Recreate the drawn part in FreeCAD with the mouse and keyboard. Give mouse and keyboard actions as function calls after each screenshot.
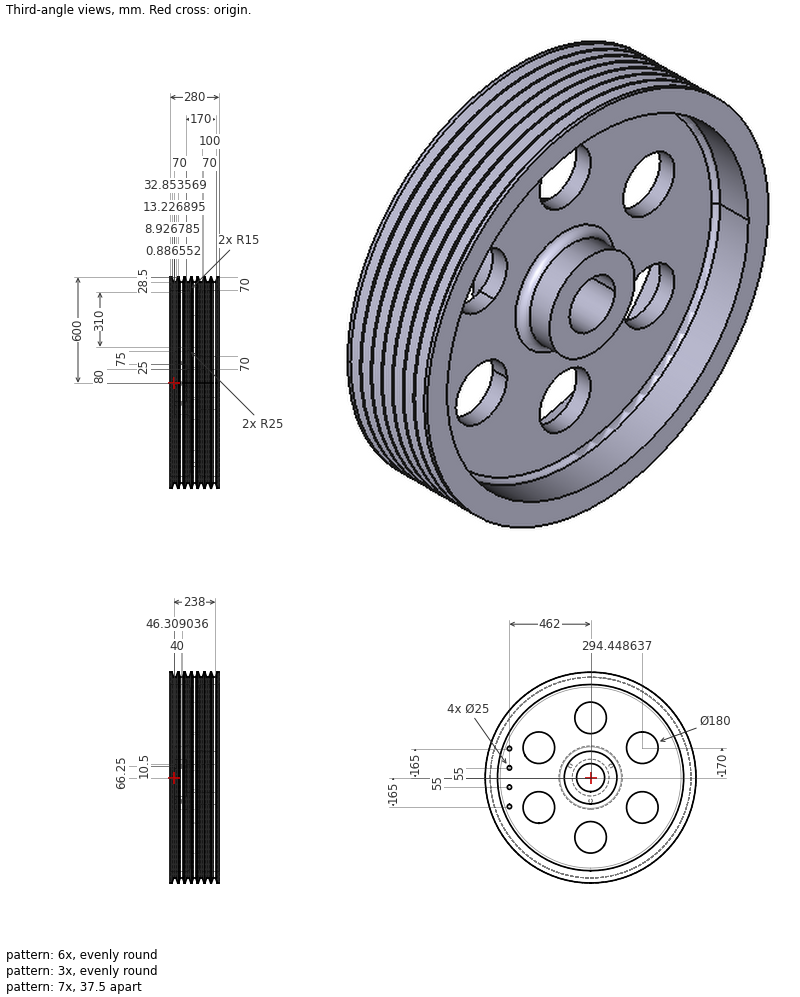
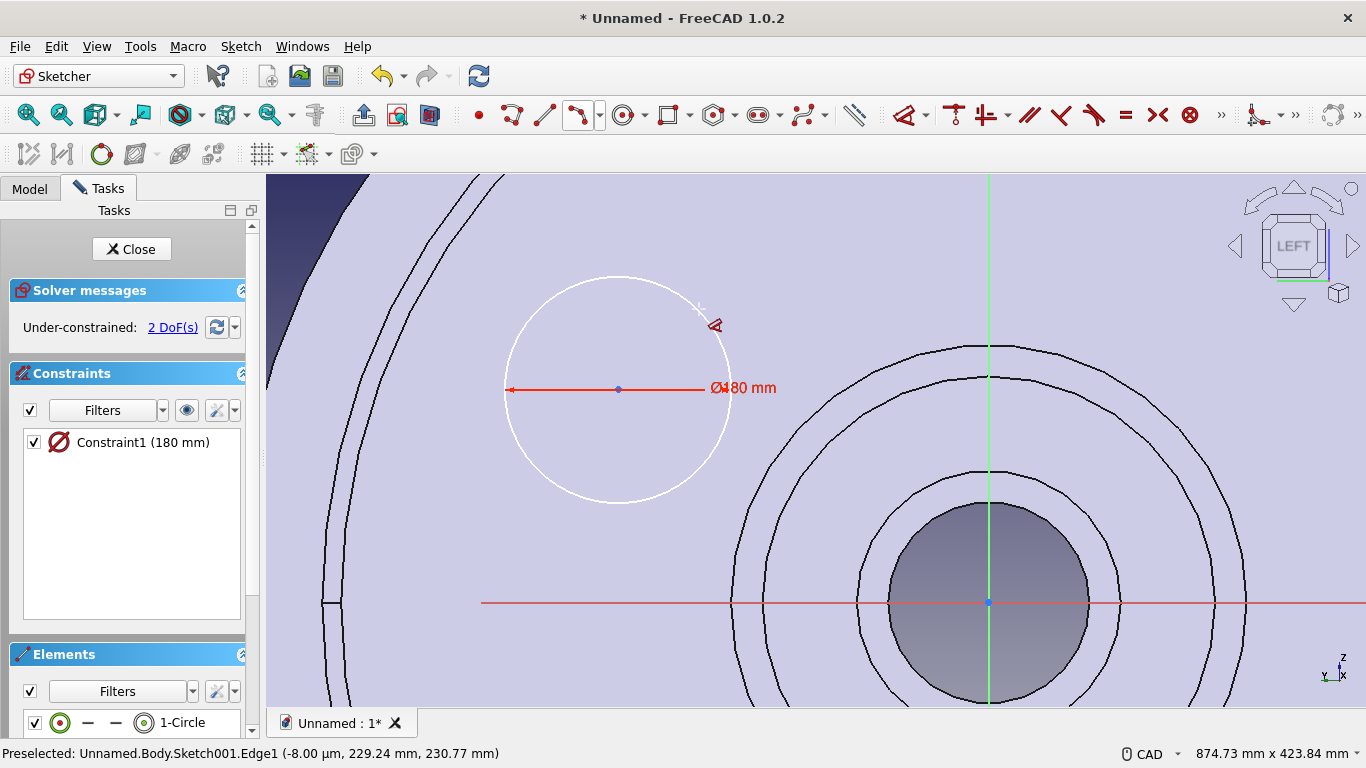
click(618, 390)
click(1023, 496)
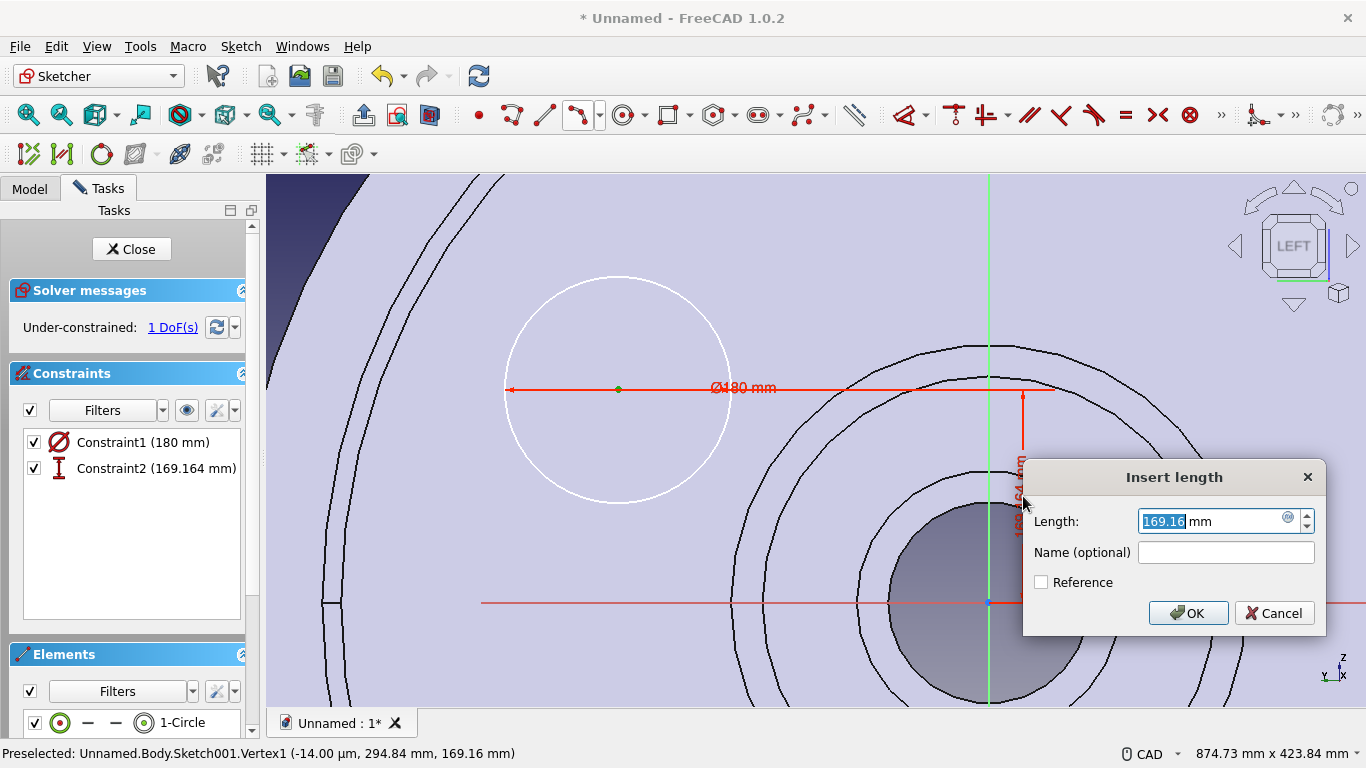
text(170)
key(Return)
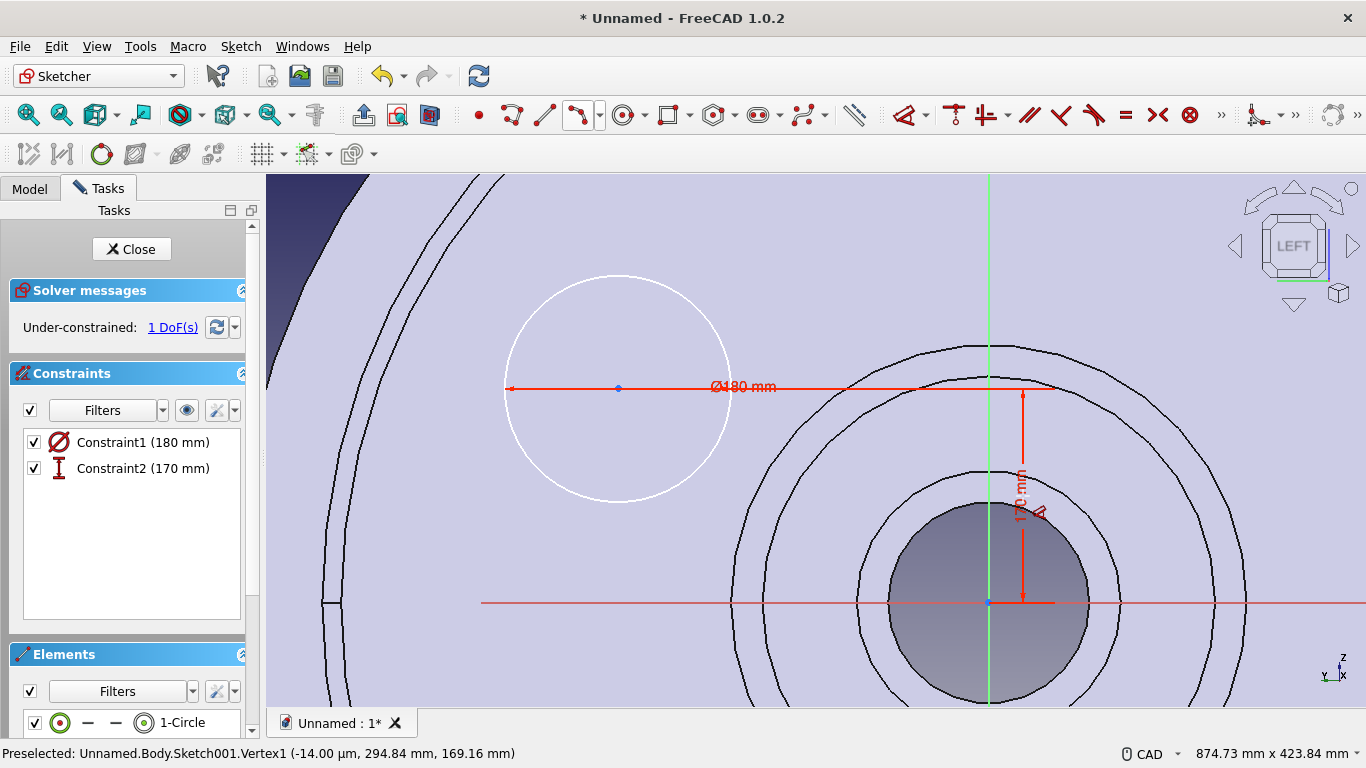
click(618, 389)
click(803, 637)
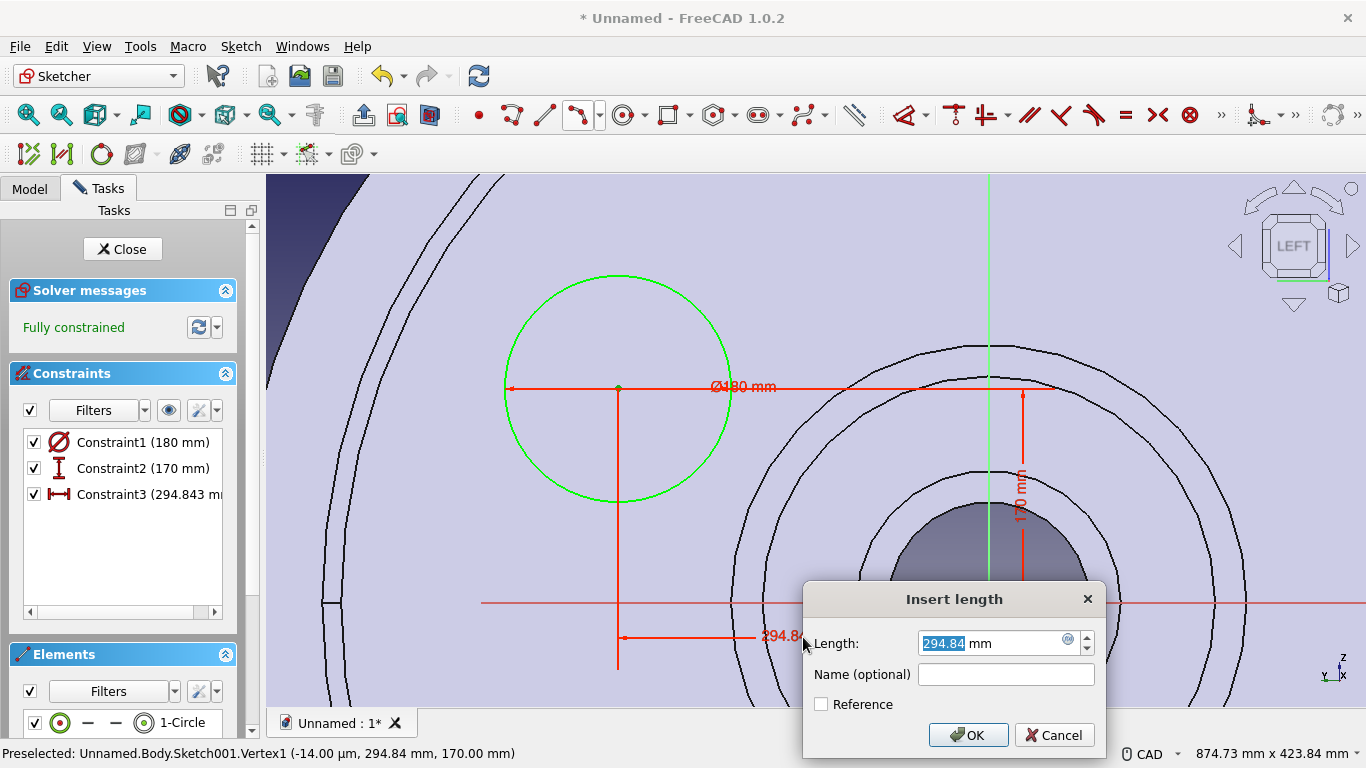
text(294.448637)
key(Return)
key(Escape)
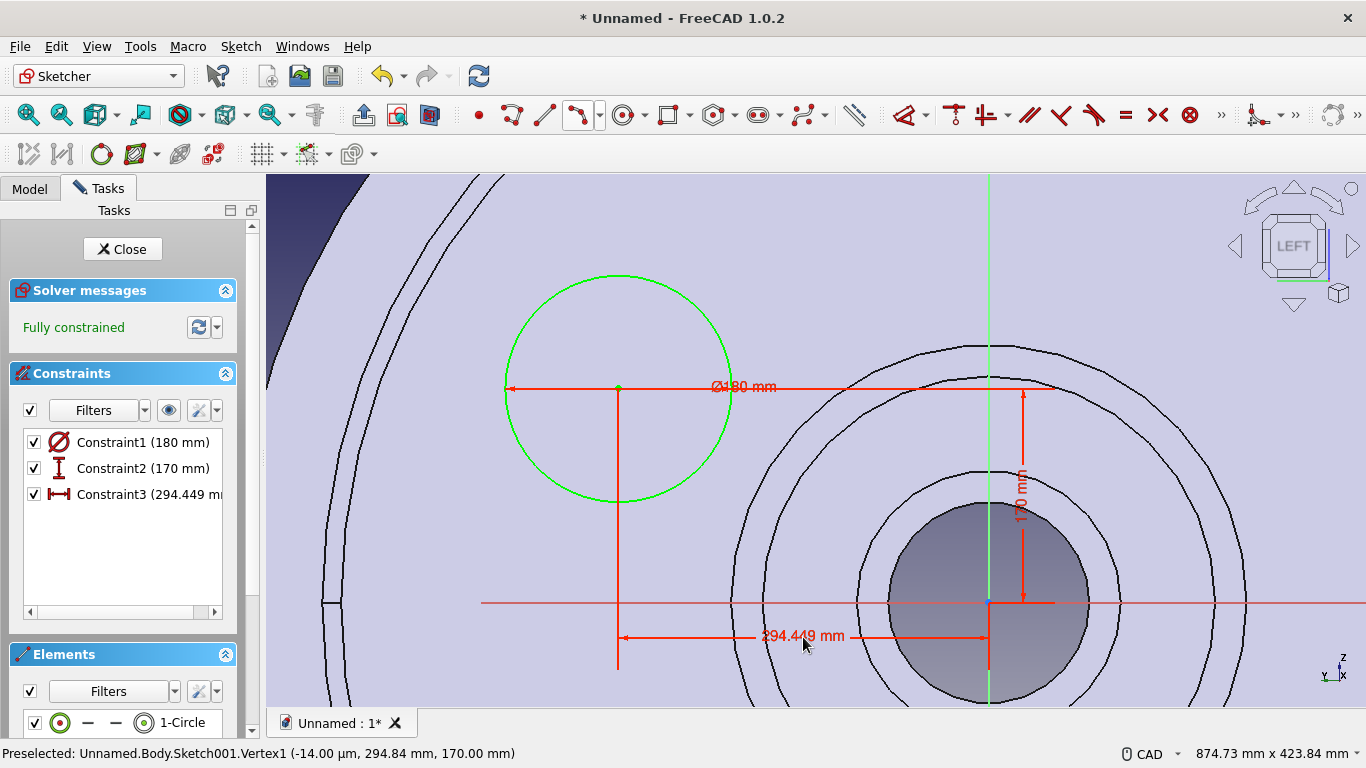
click(123, 249)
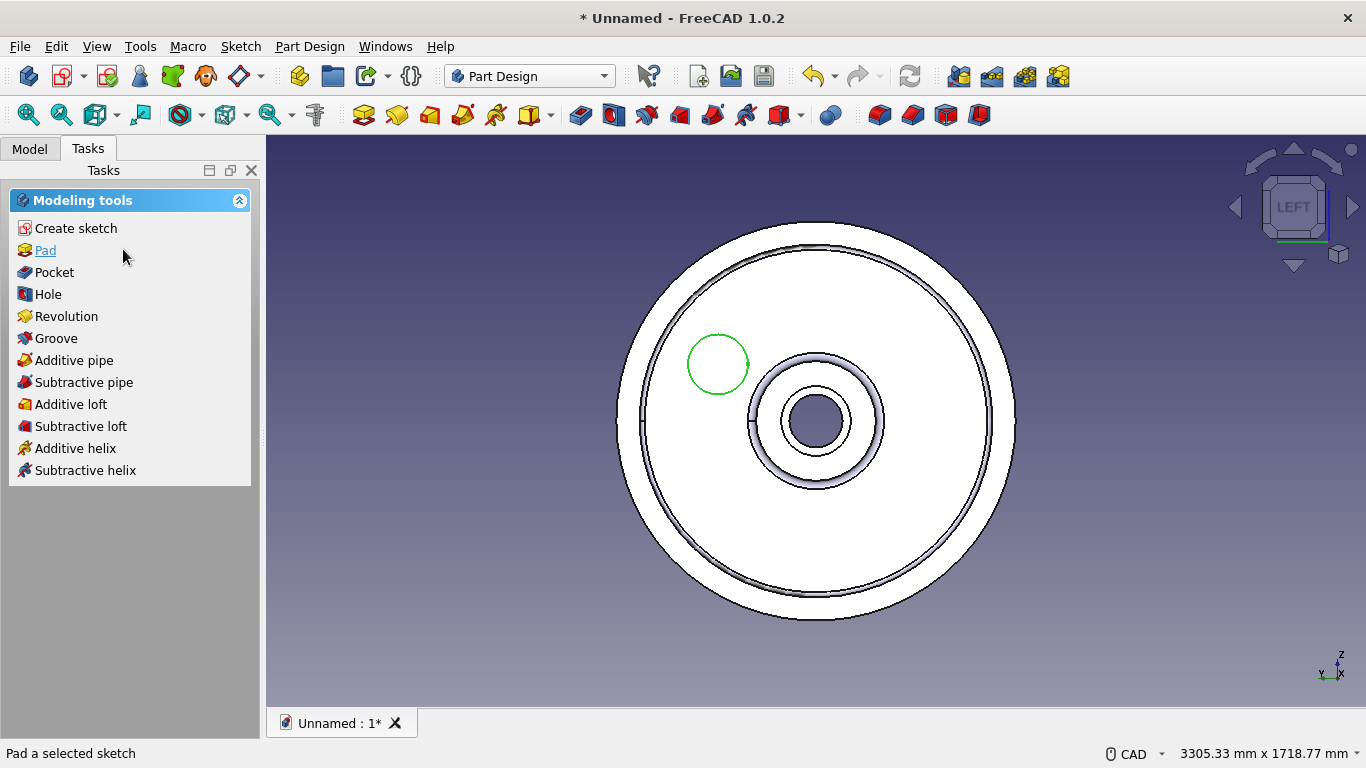
click(581, 116)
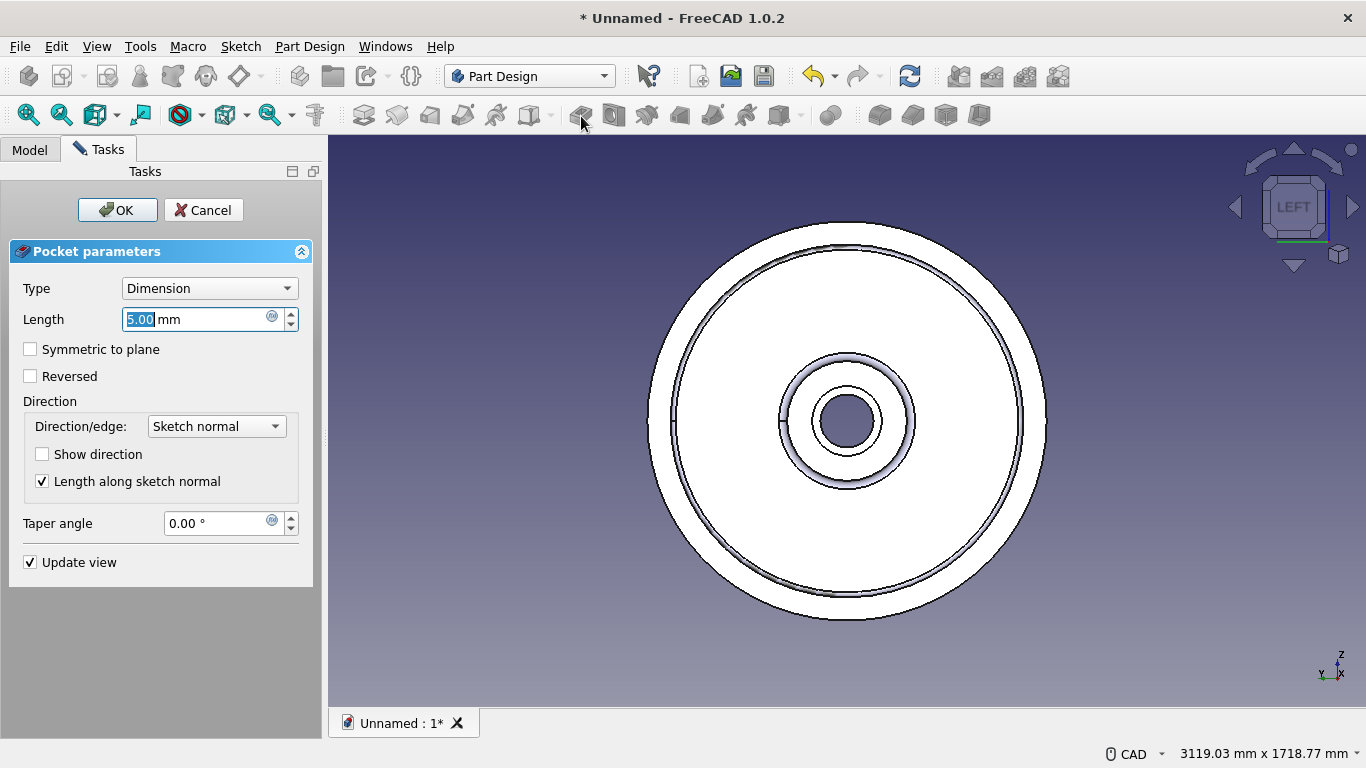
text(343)
key(Tab)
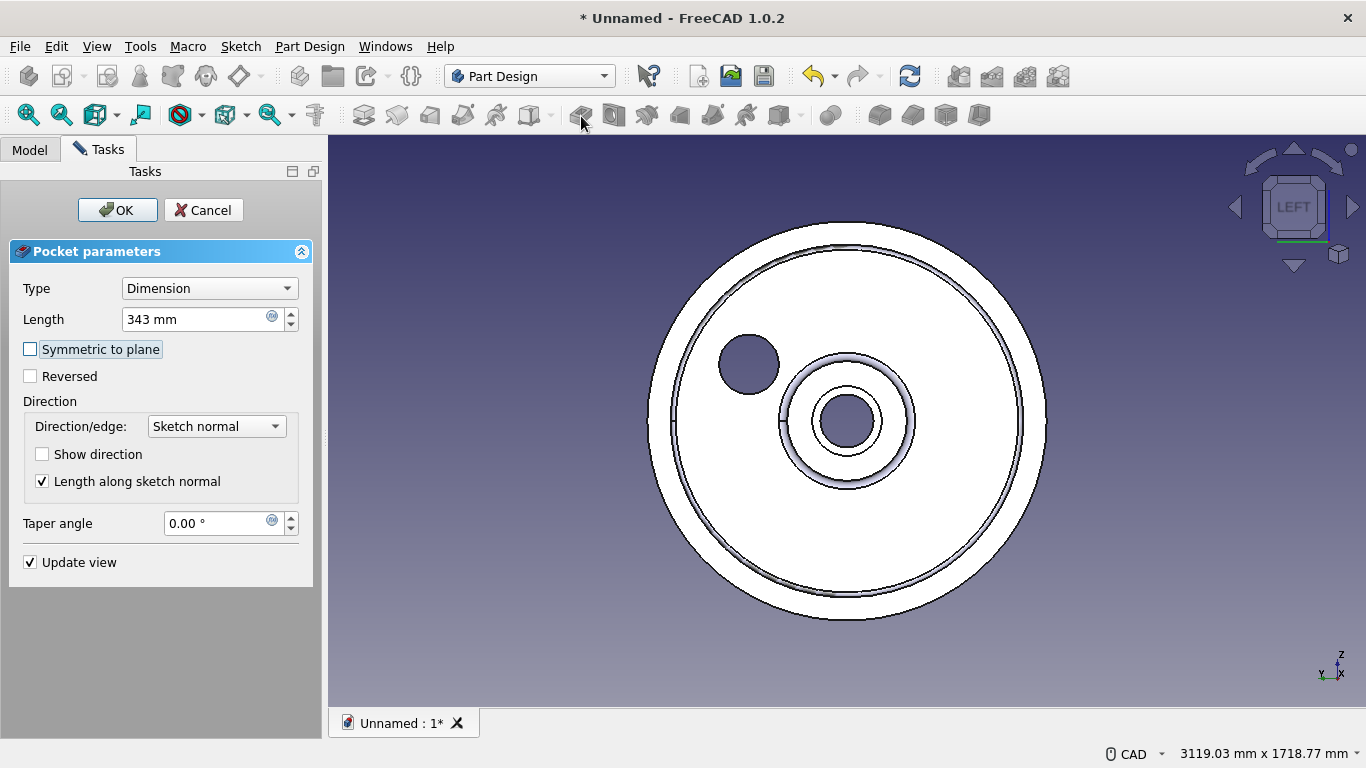
click(118, 210)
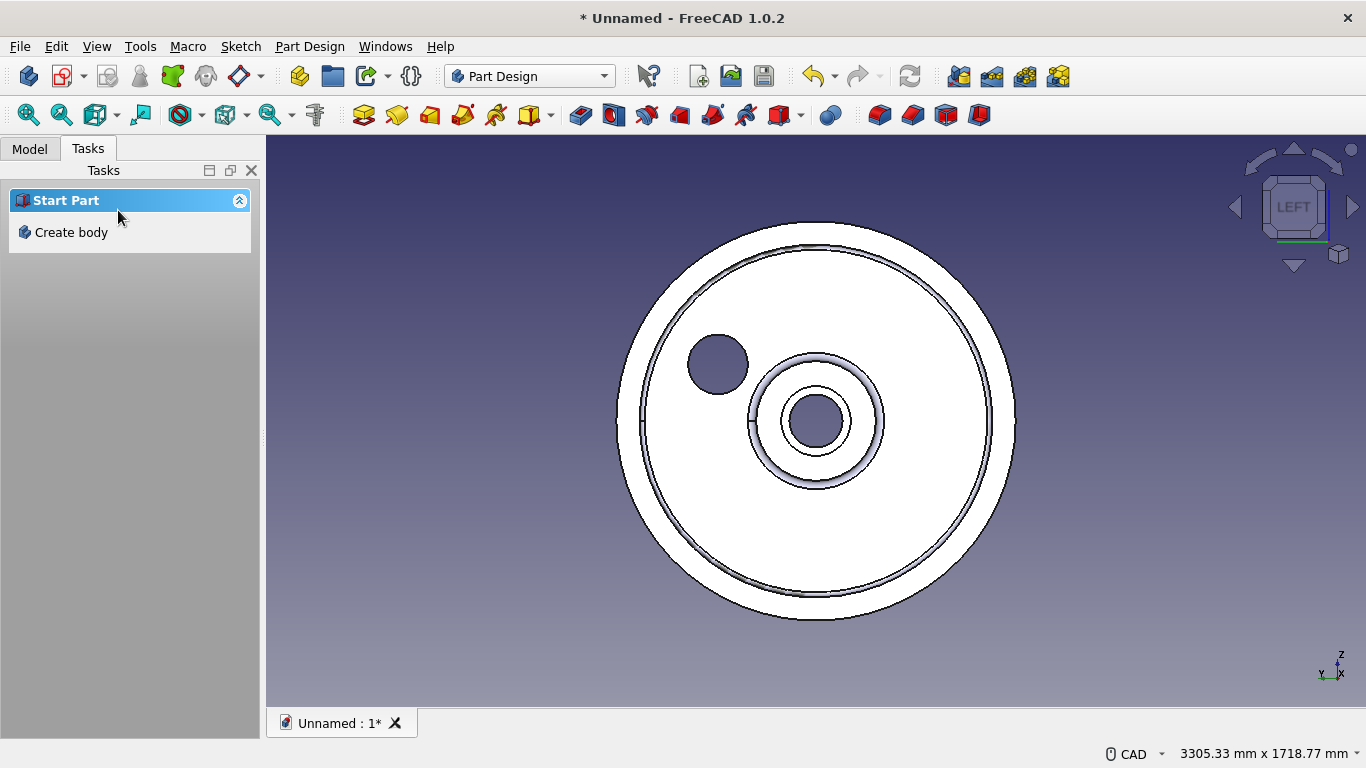
click(30, 148)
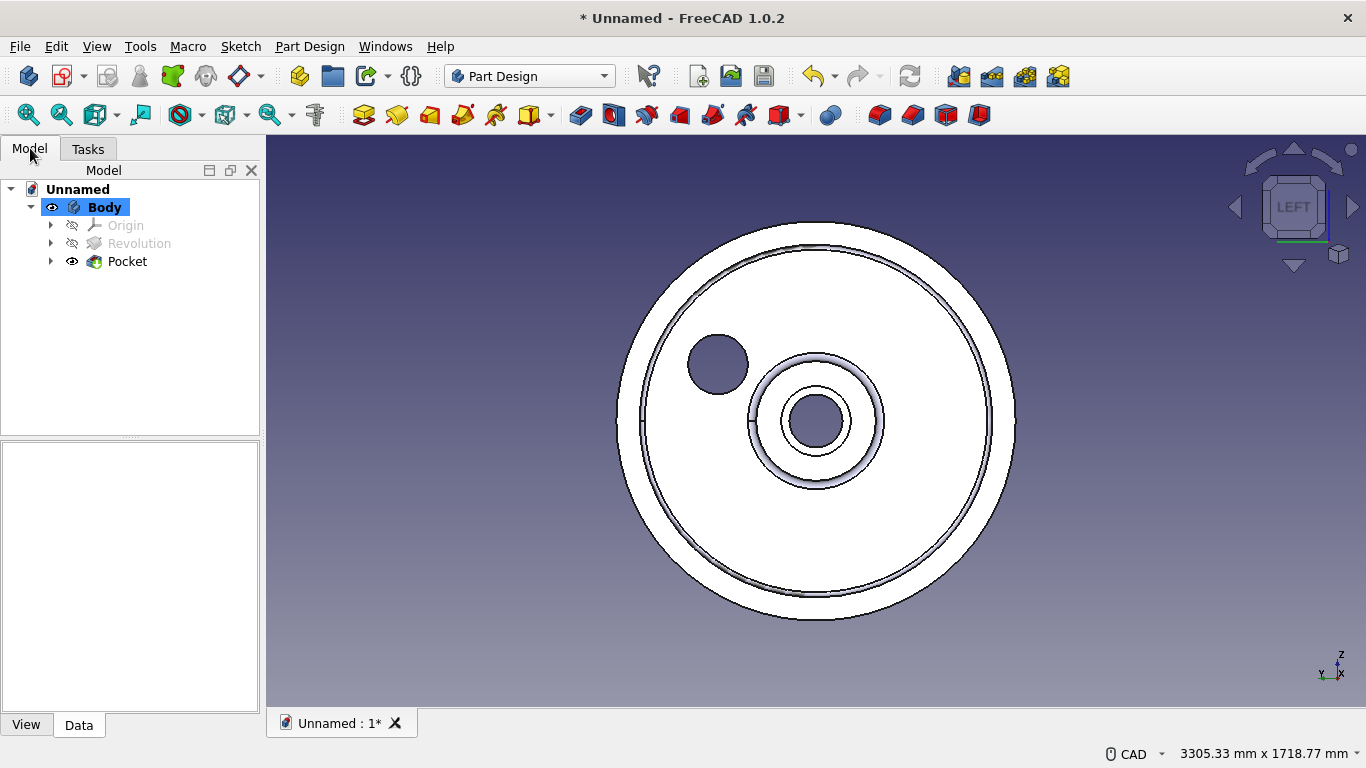
click(117, 261)